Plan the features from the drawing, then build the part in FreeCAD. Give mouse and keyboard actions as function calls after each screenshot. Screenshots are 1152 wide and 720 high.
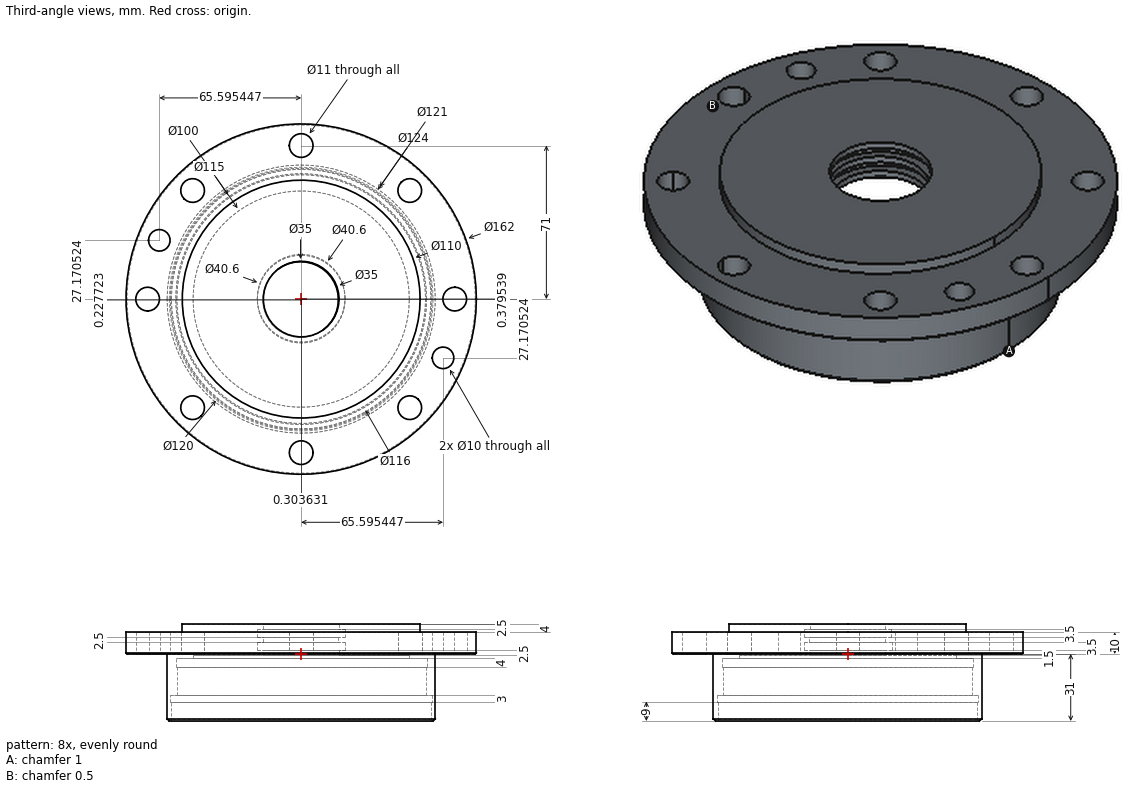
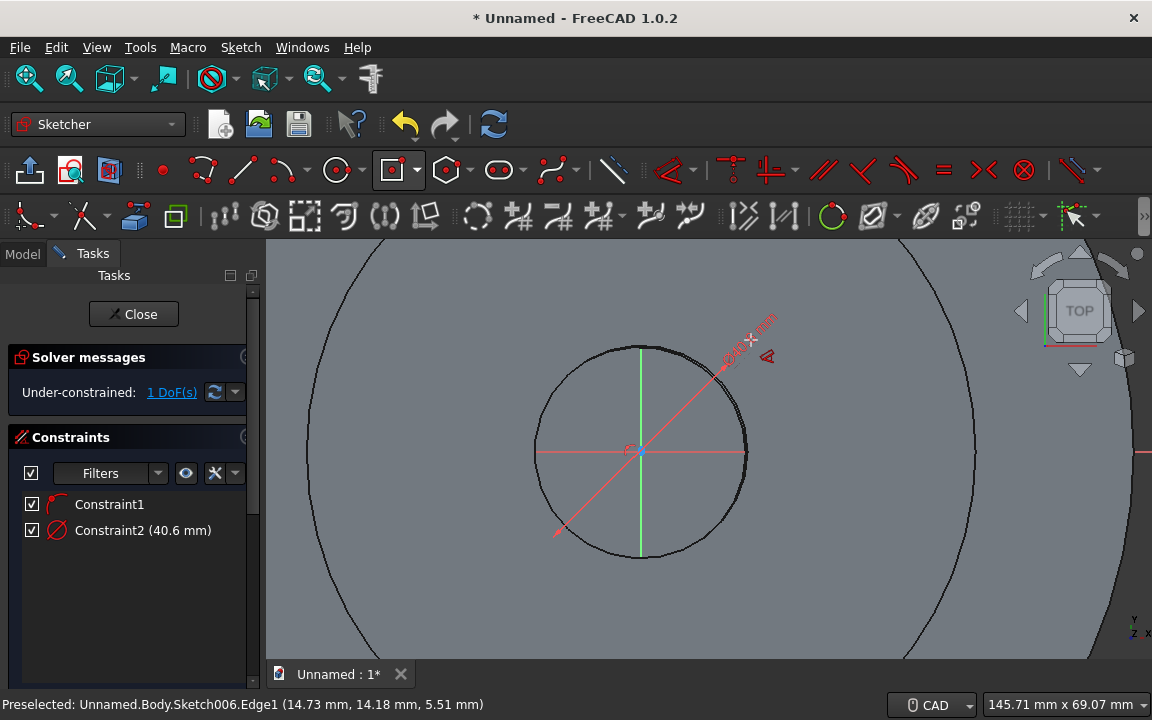
scroll(641, 450, up, 15)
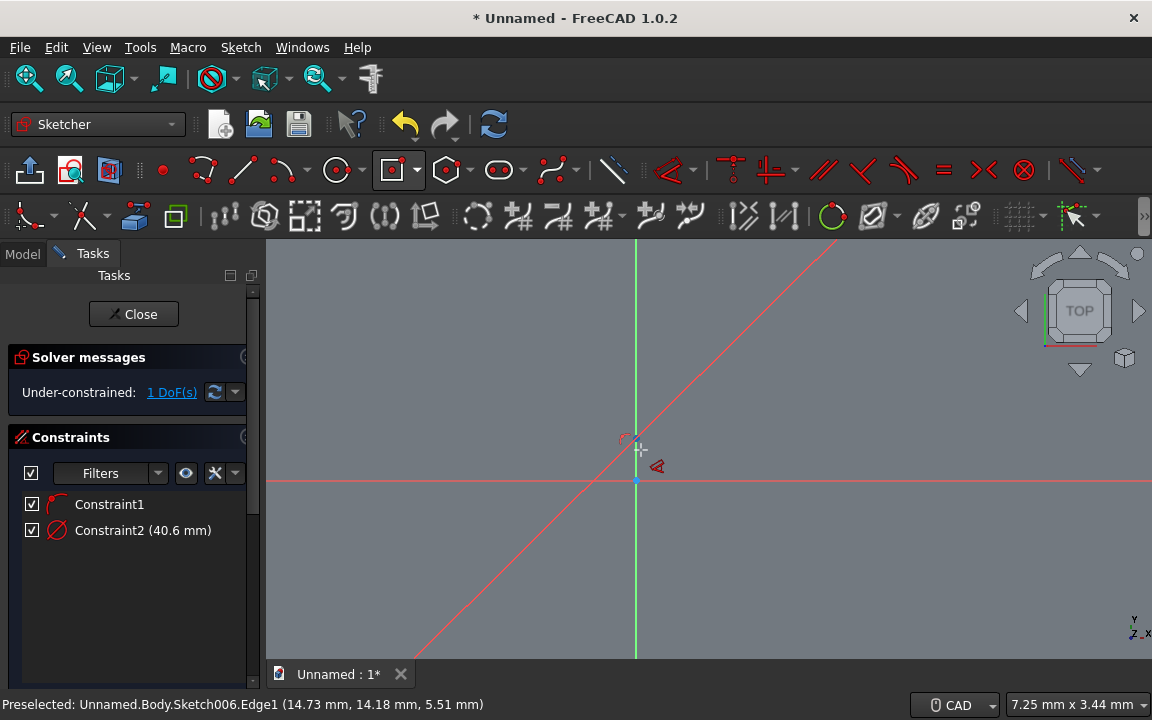
click(636, 438)
click(670, 459)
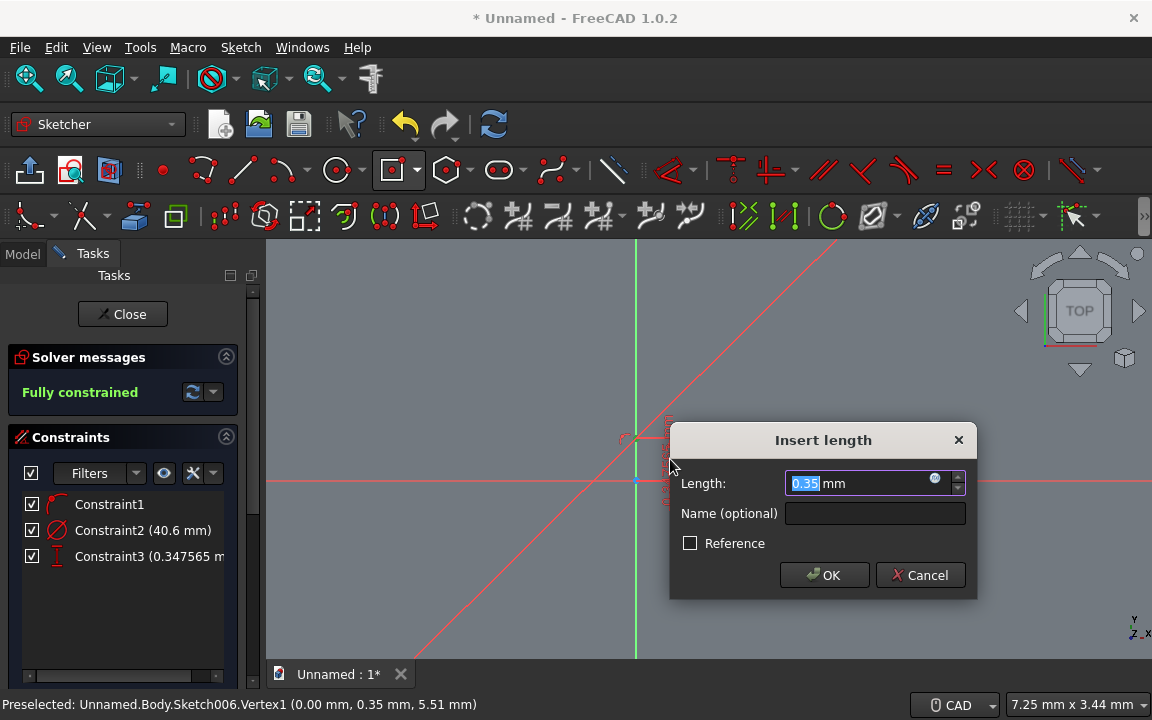
text(0.379539)
key(Return)
key(Escape)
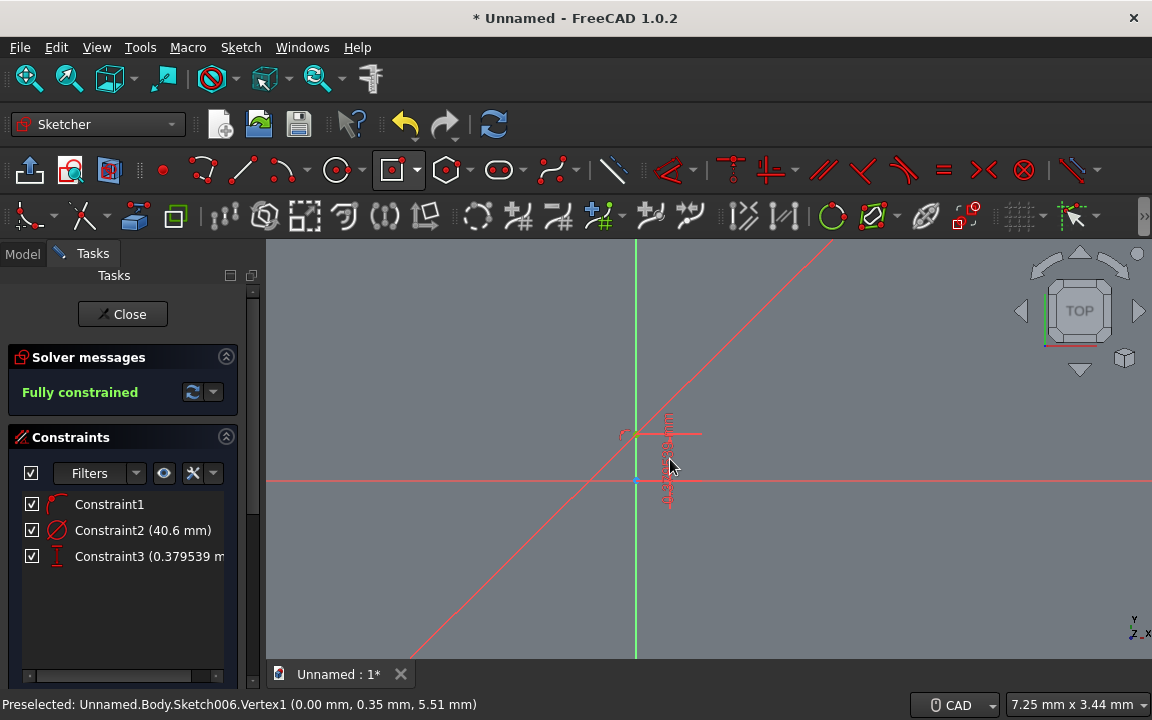
click(123, 314)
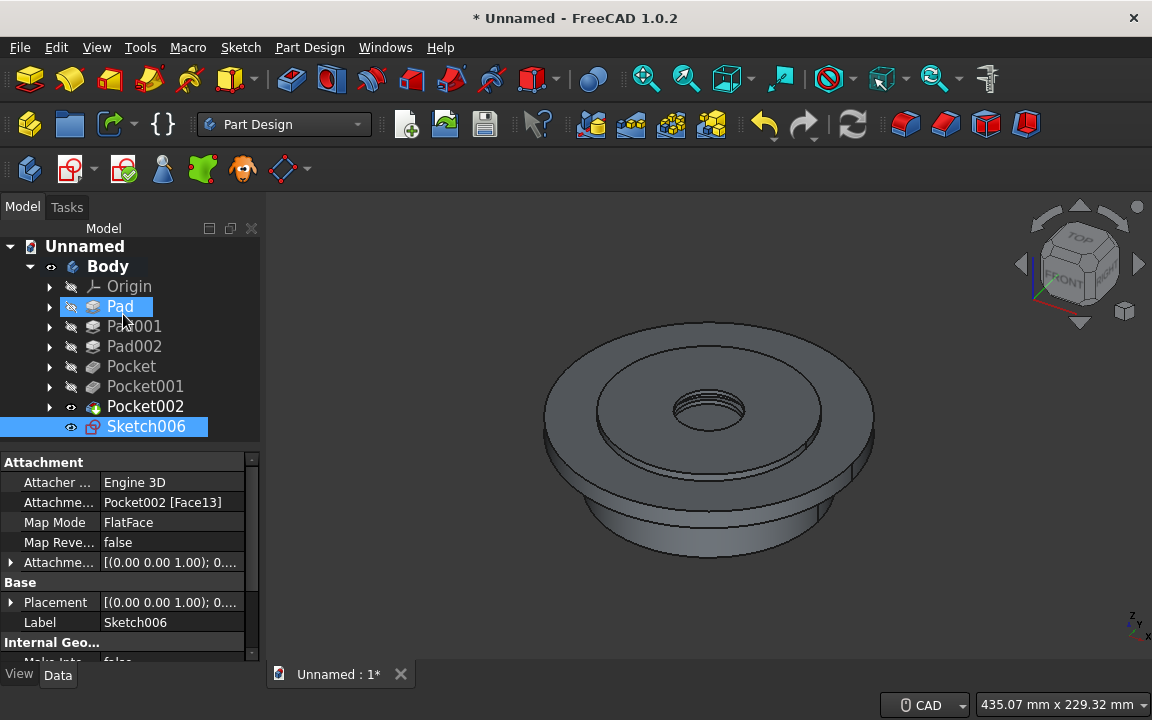
click(292, 80)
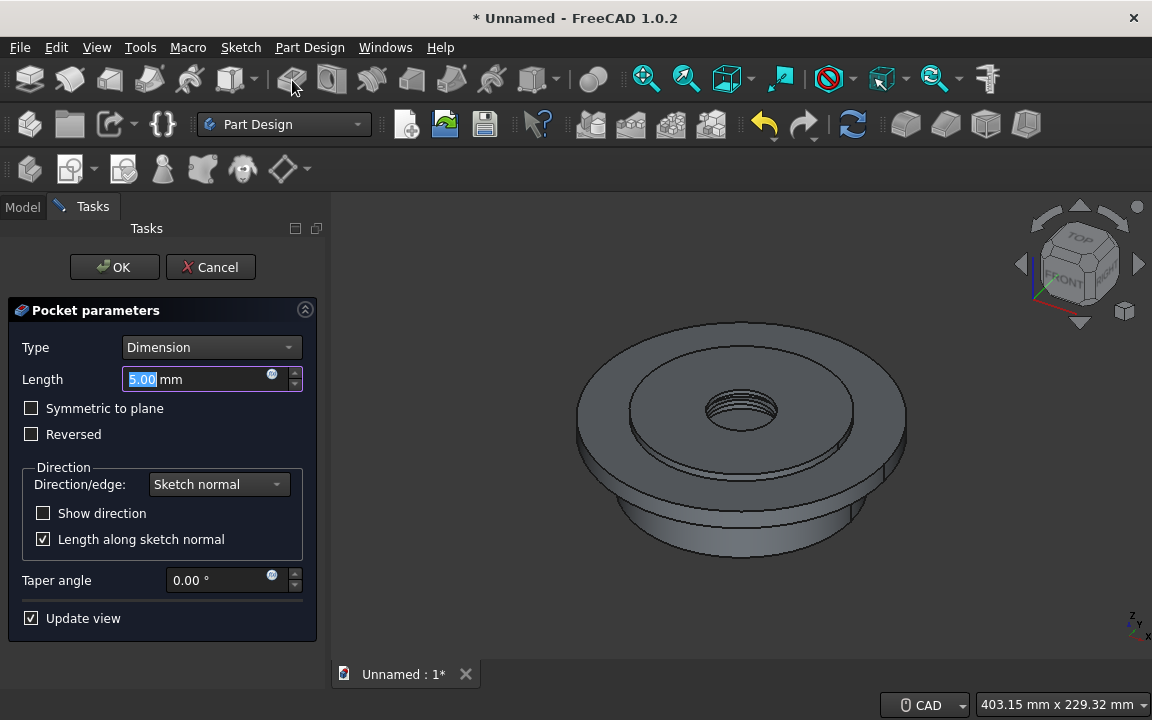
text(3.5)
key(Tab)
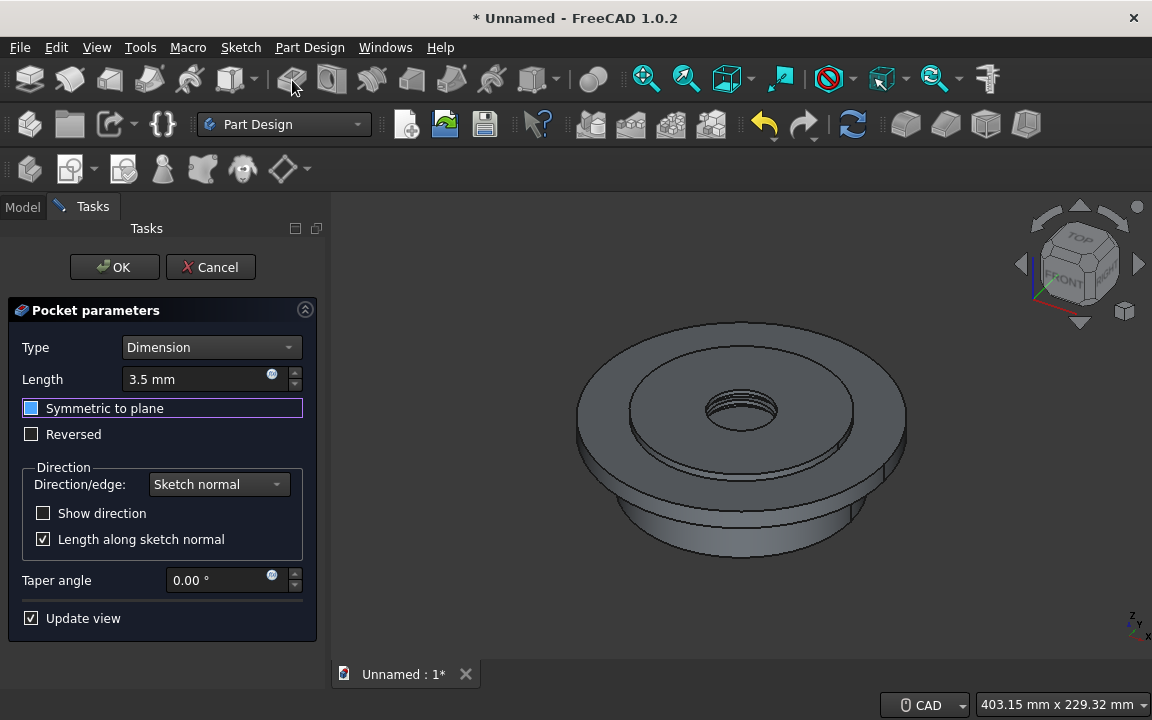
click(115, 267)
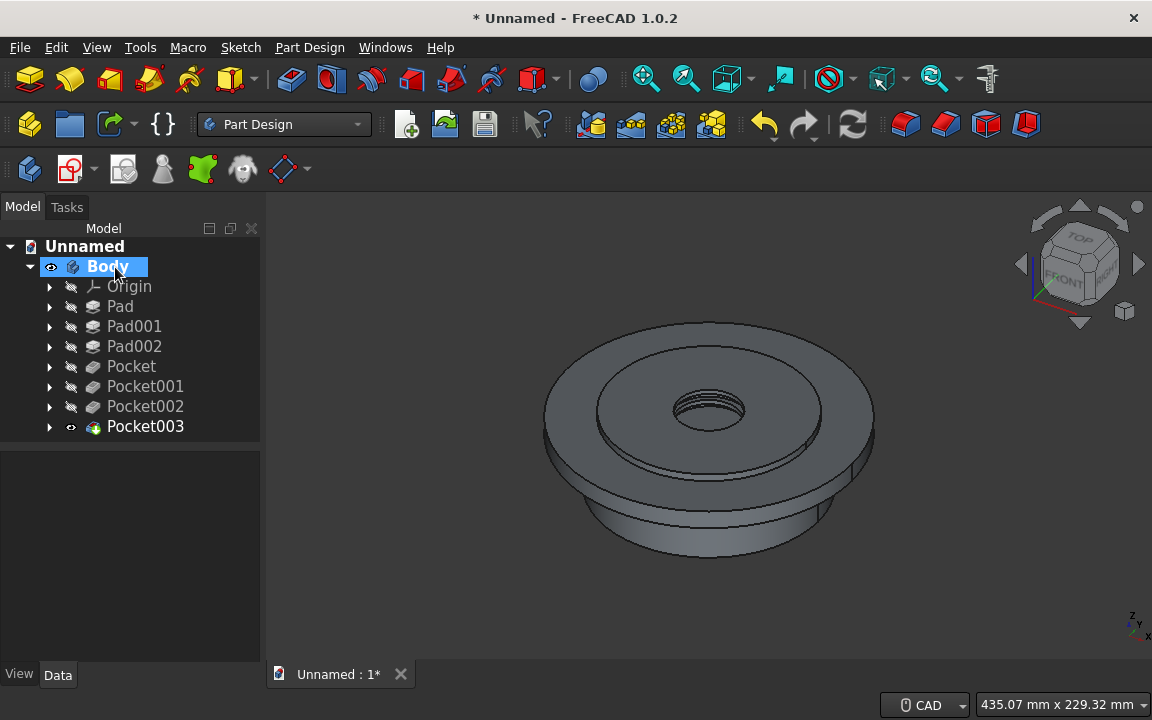
click(705, 420)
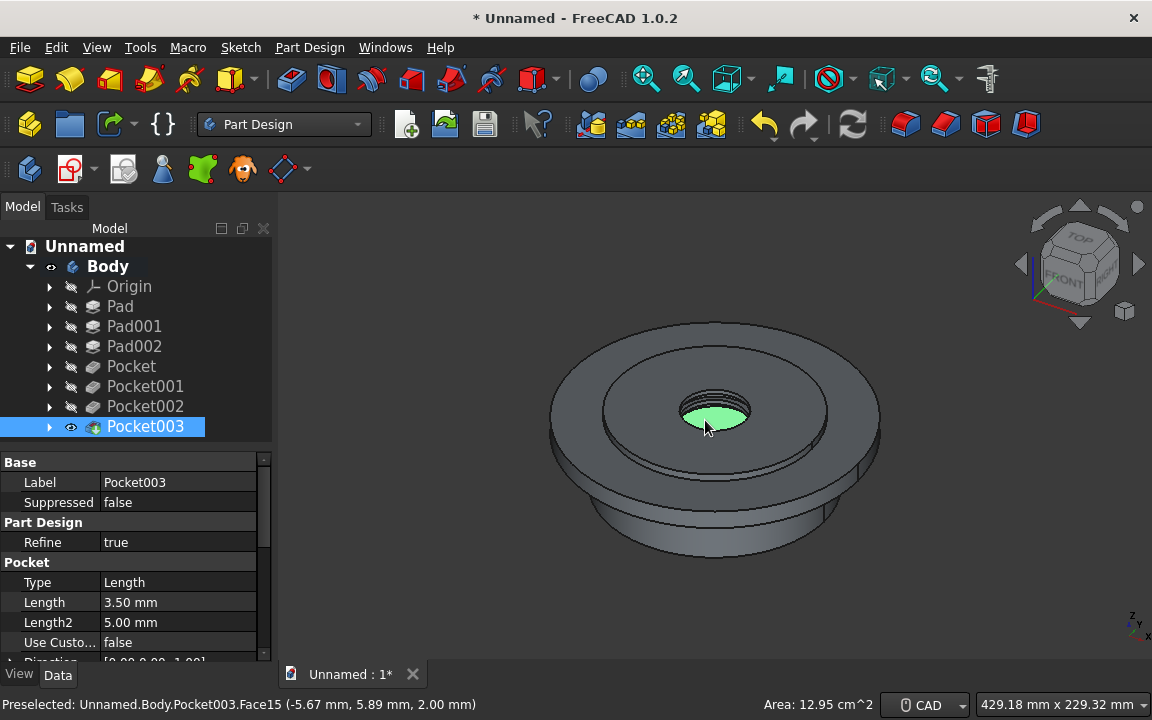
click(70, 170)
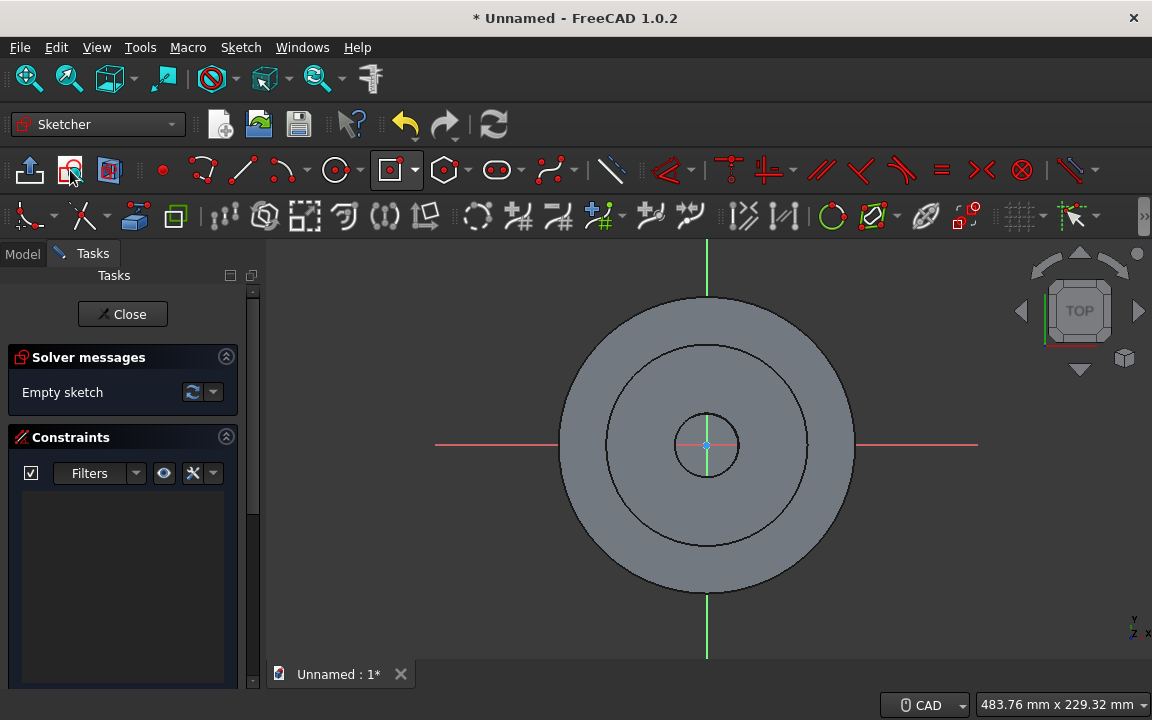
click(110, 170)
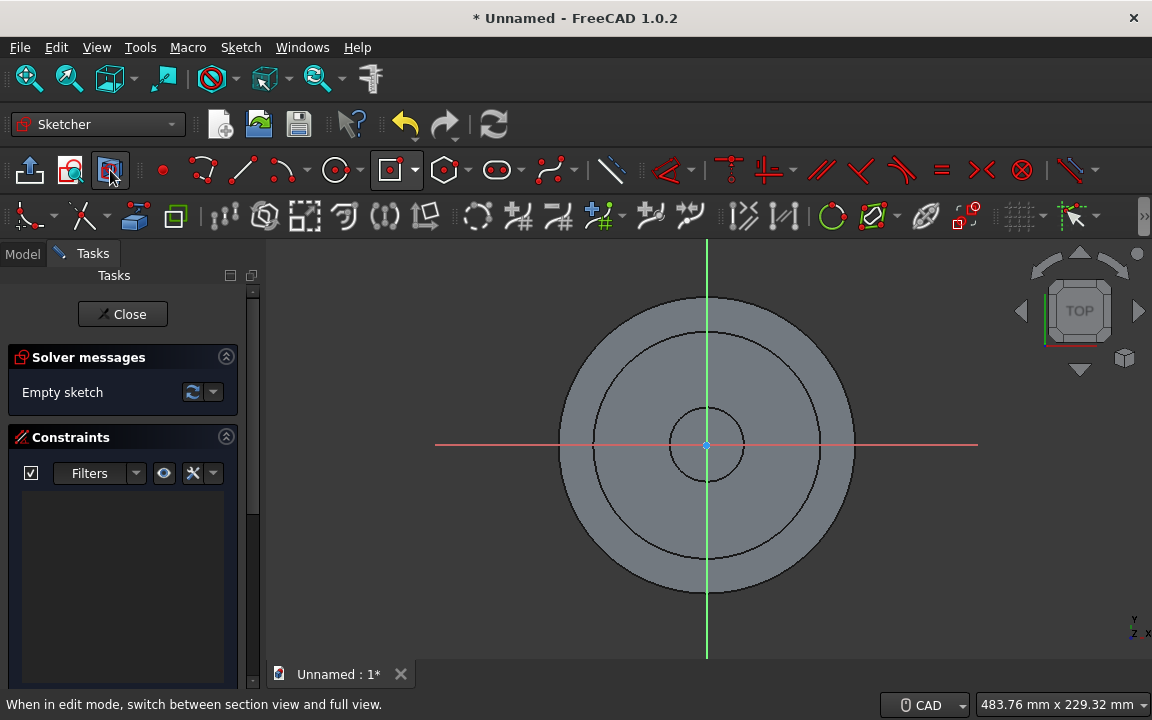
scroll(729, 444, up, 7)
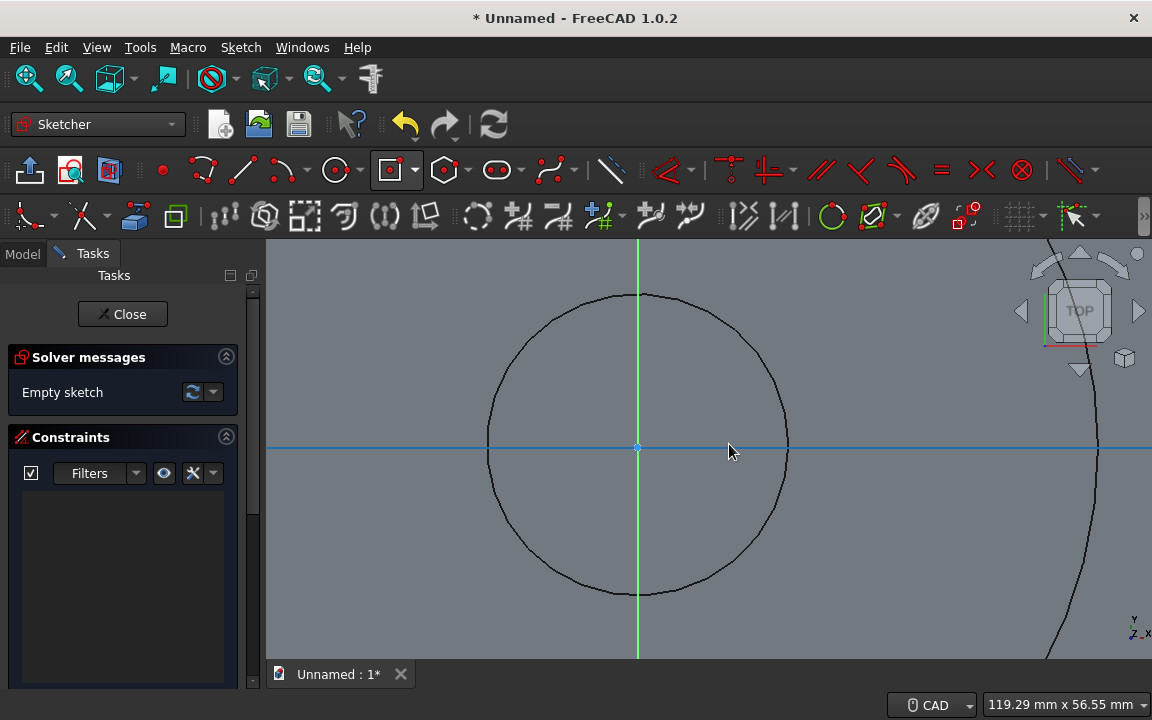
click(336, 170)